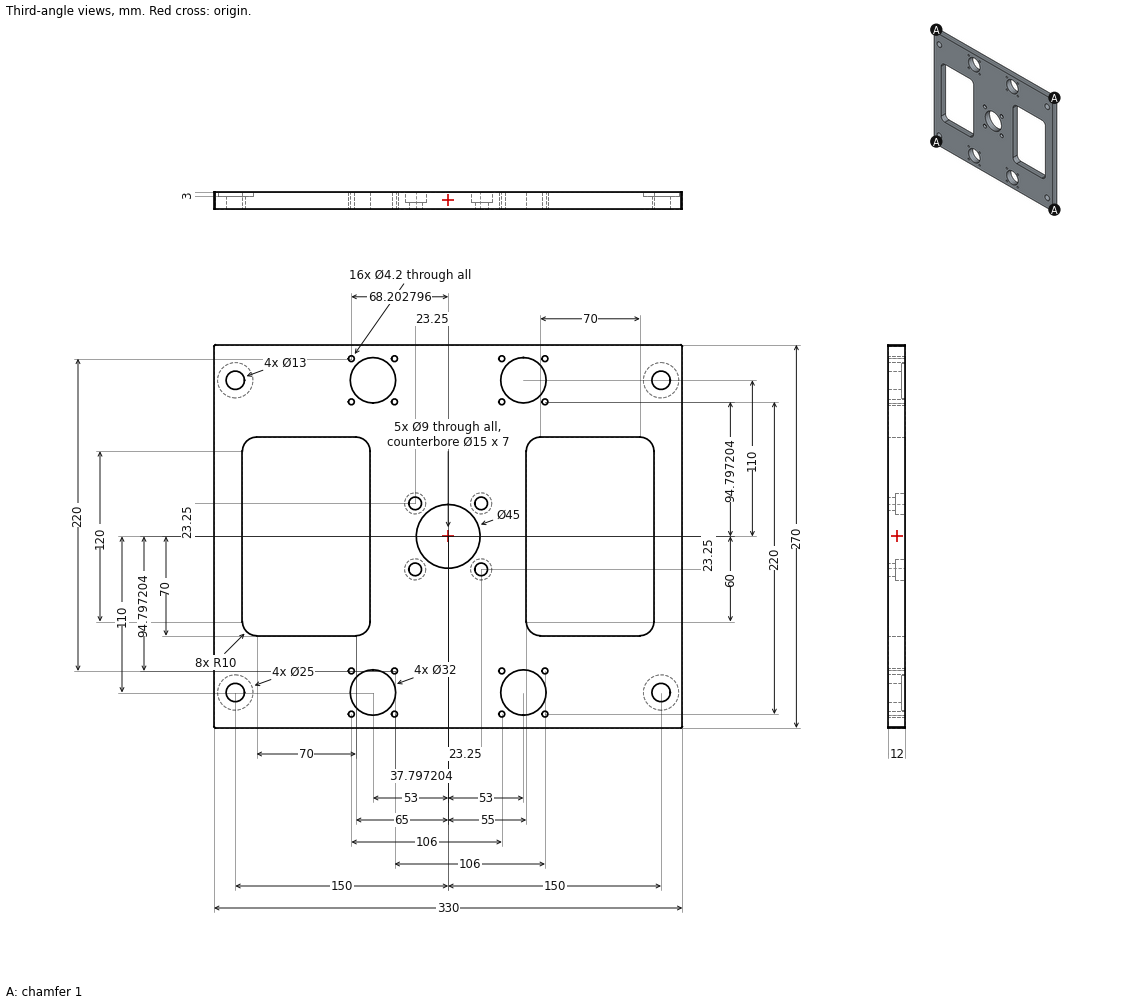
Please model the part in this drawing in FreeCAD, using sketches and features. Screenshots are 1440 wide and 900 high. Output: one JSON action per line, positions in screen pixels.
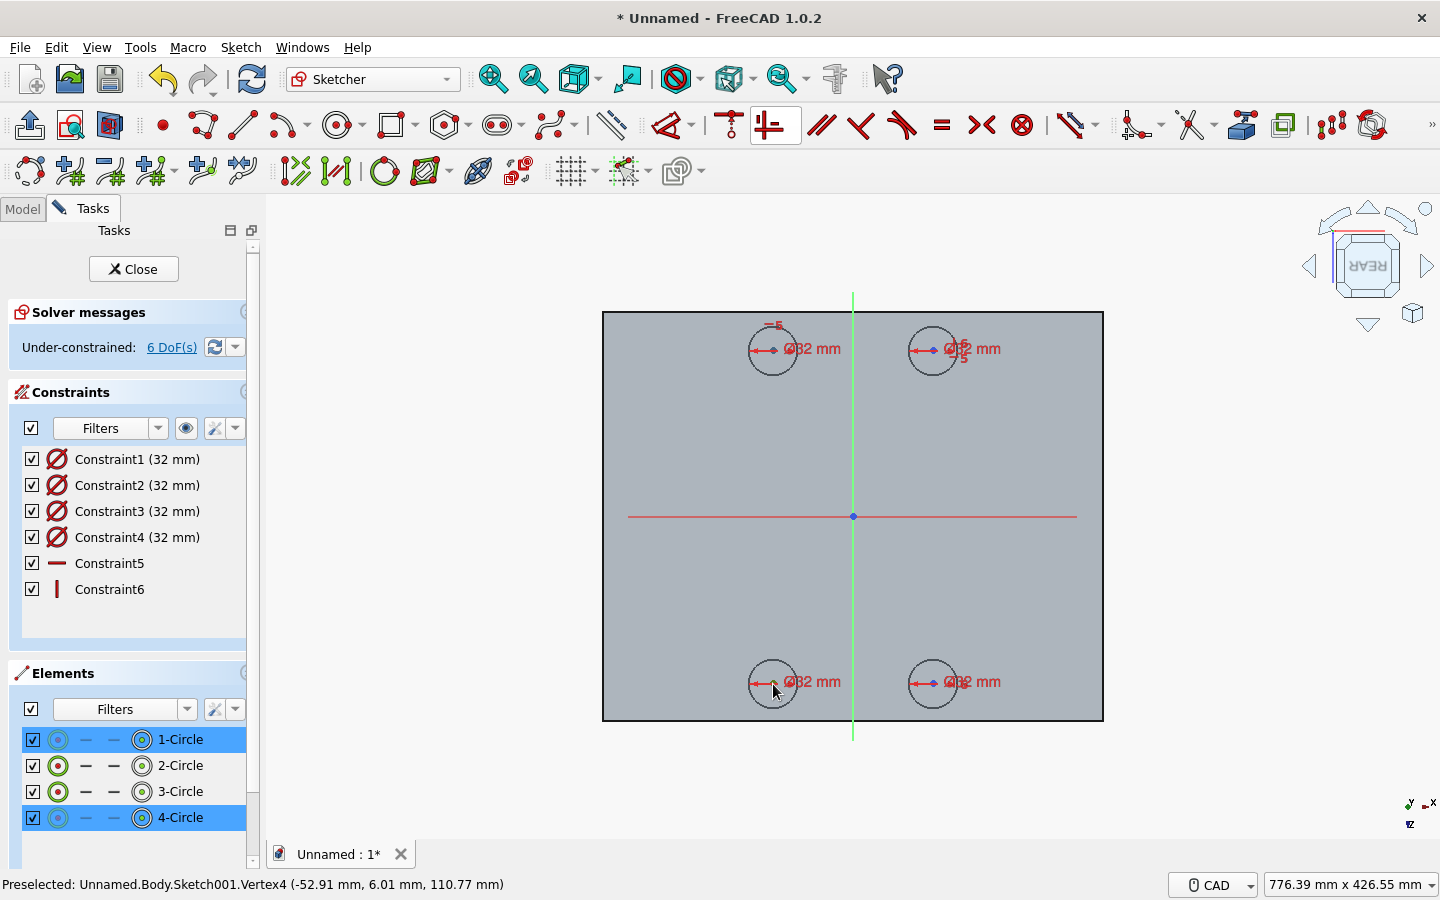
{"action": "left_click", "coordinate": [796, 126]}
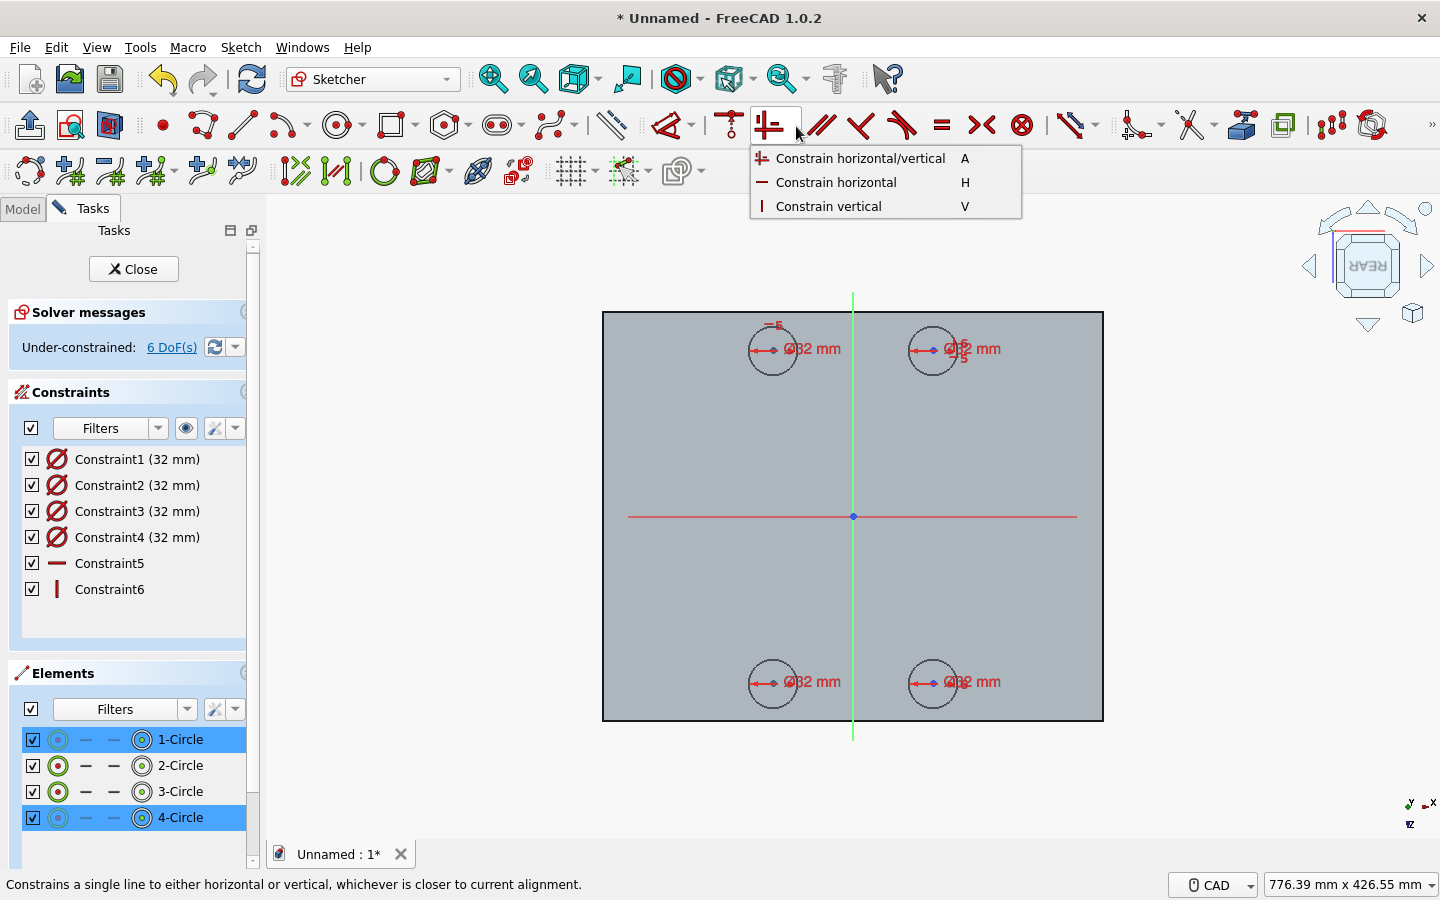
{"action": "left_click", "coordinate": [886, 206]}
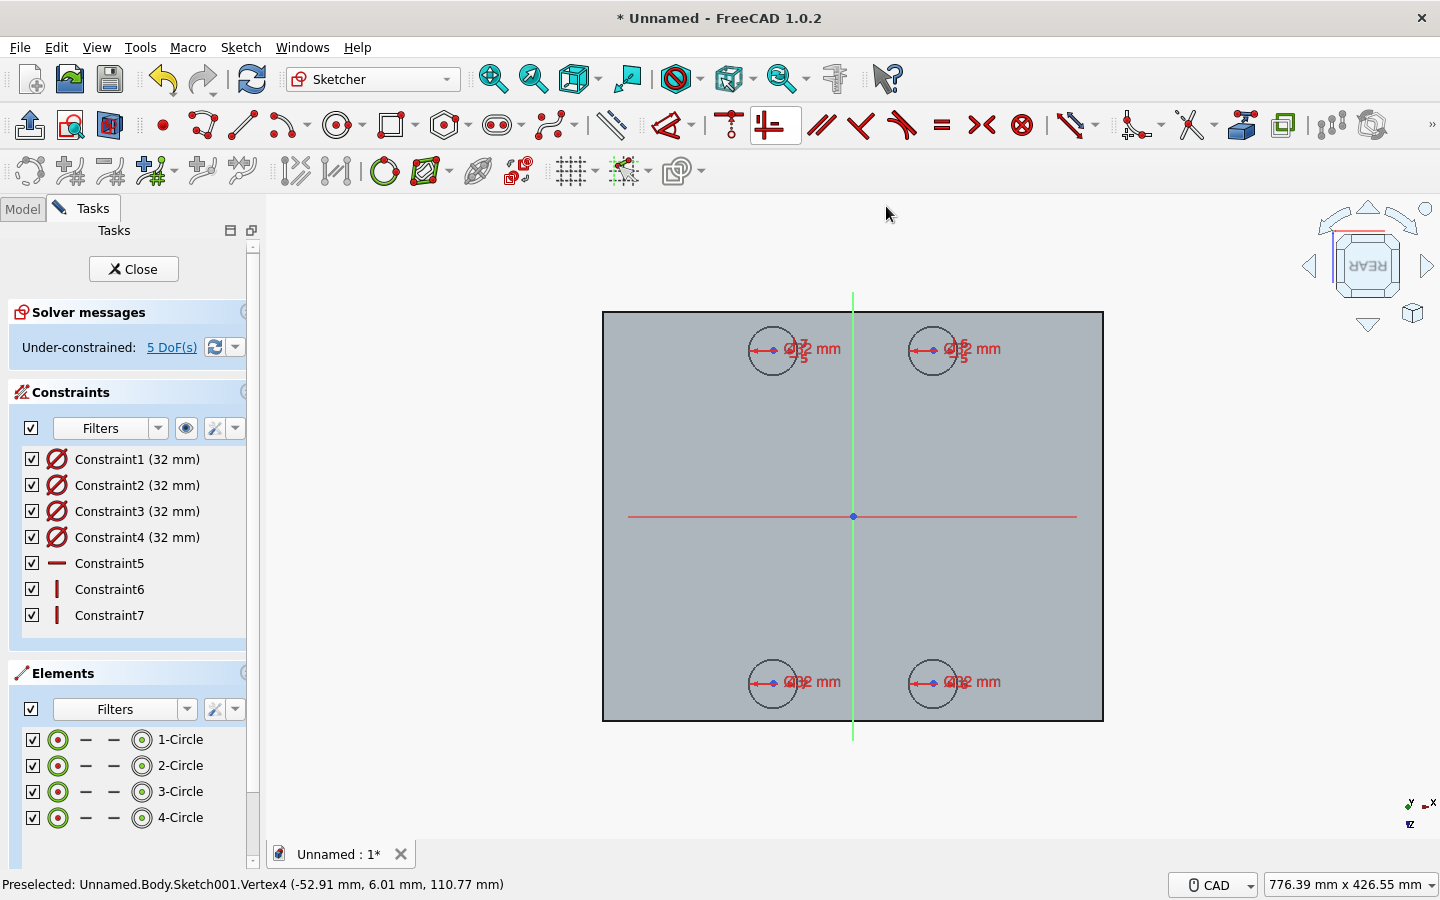
{"action": "left_click", "coordinate": [933, 684]}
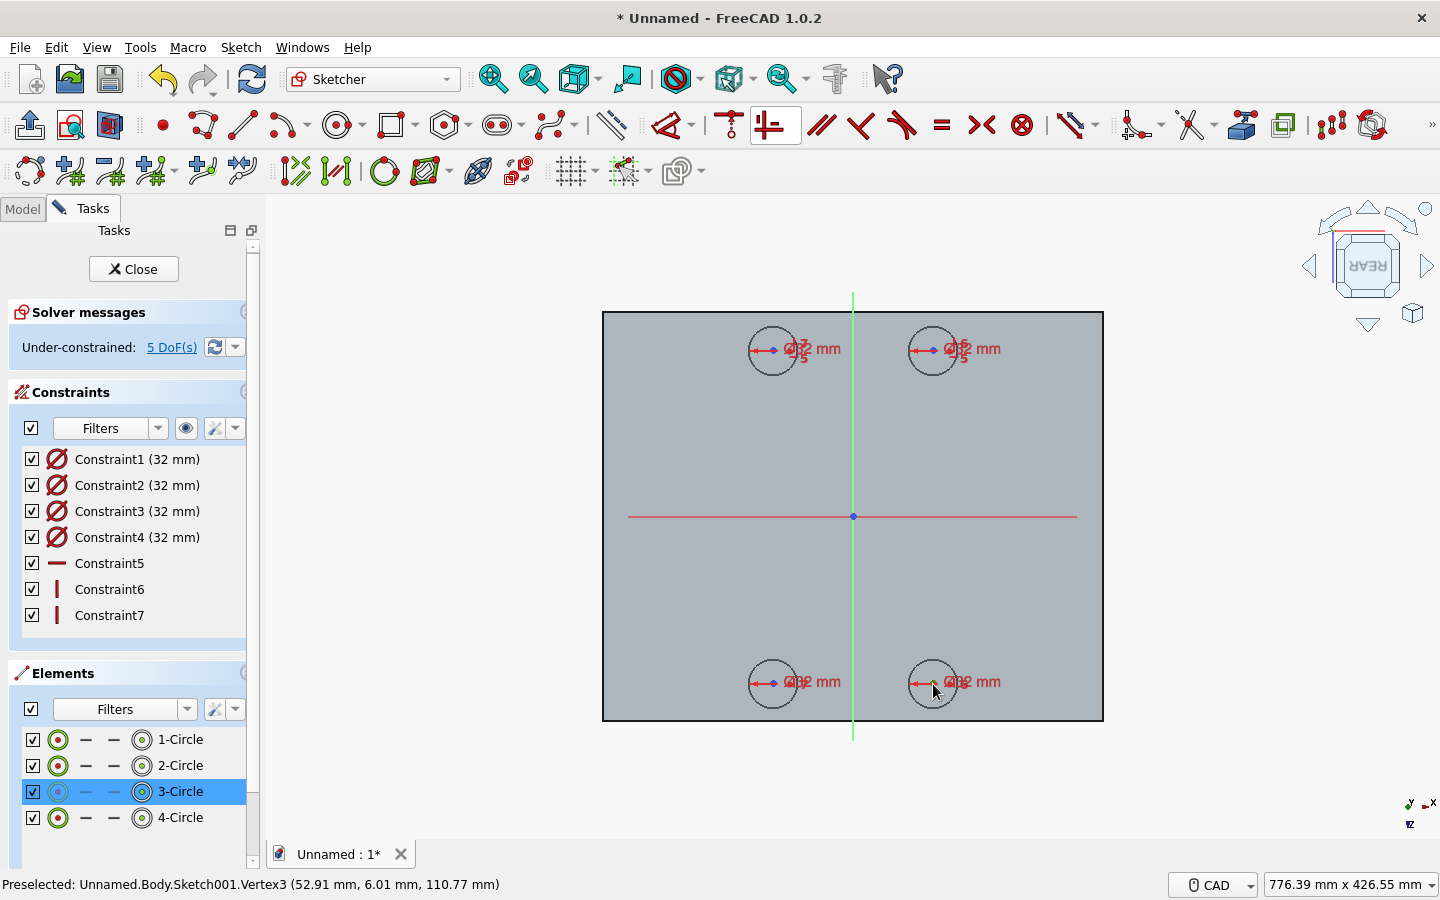
{"action": "left_click", "coordinate": [773, 684]}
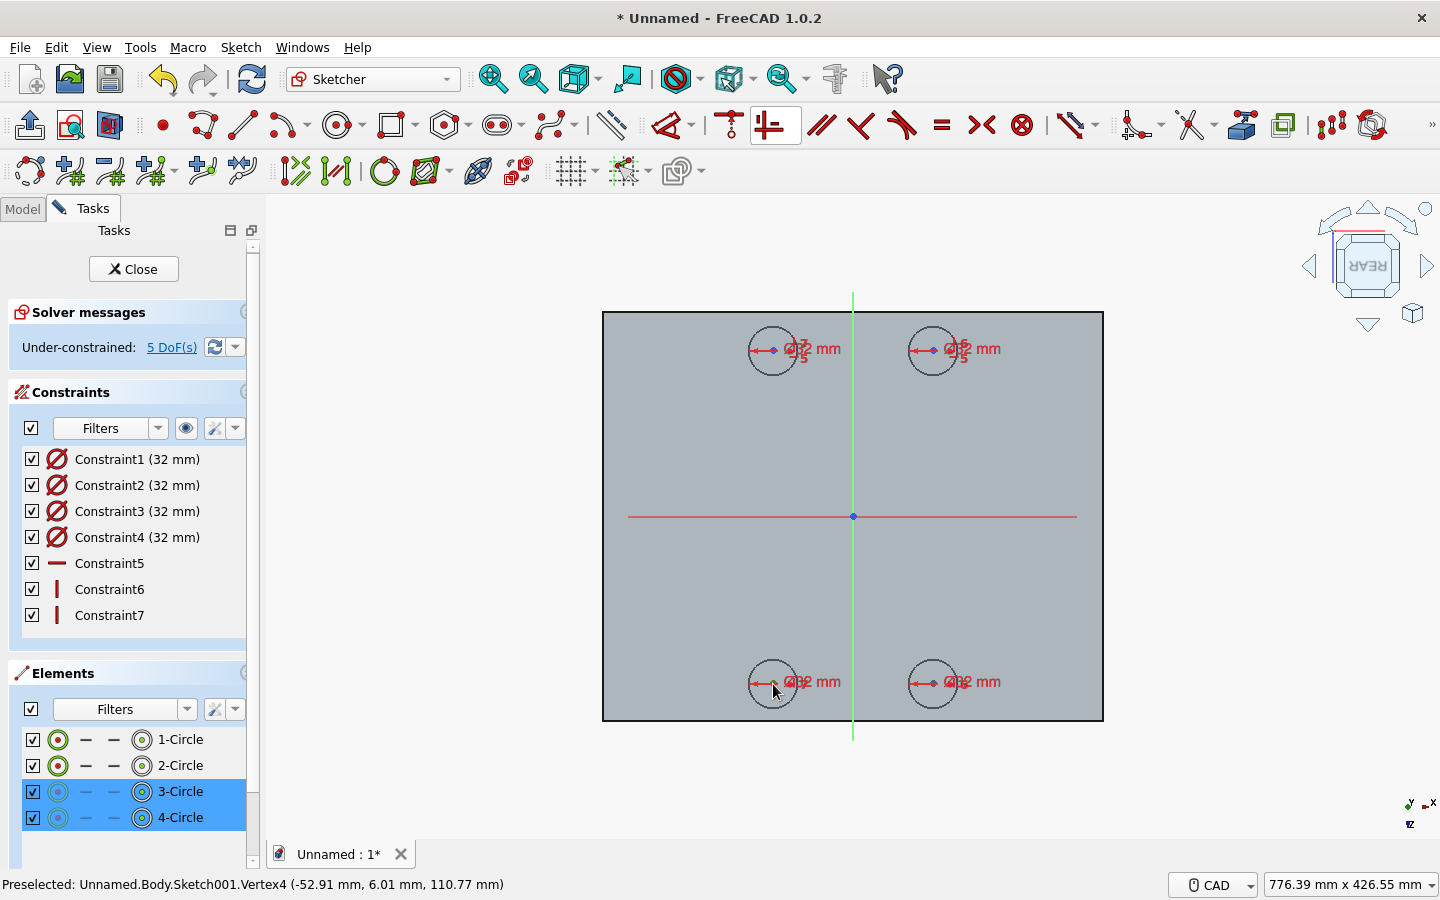
{"action": "left_click", "coordinate": [796, 126]}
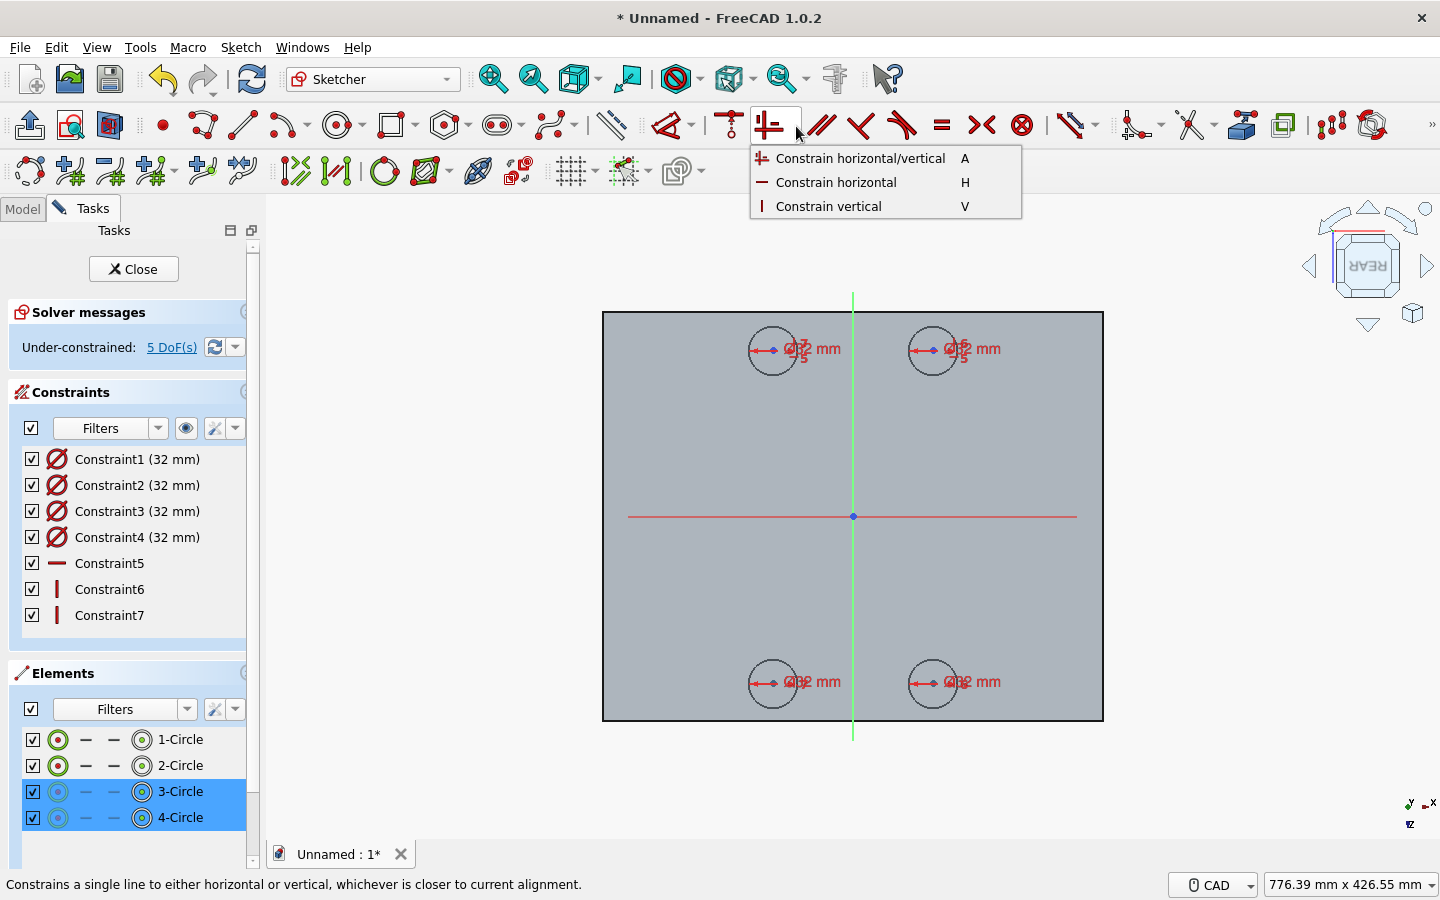
{"action": "left_click", "coordinate": [886, 182]}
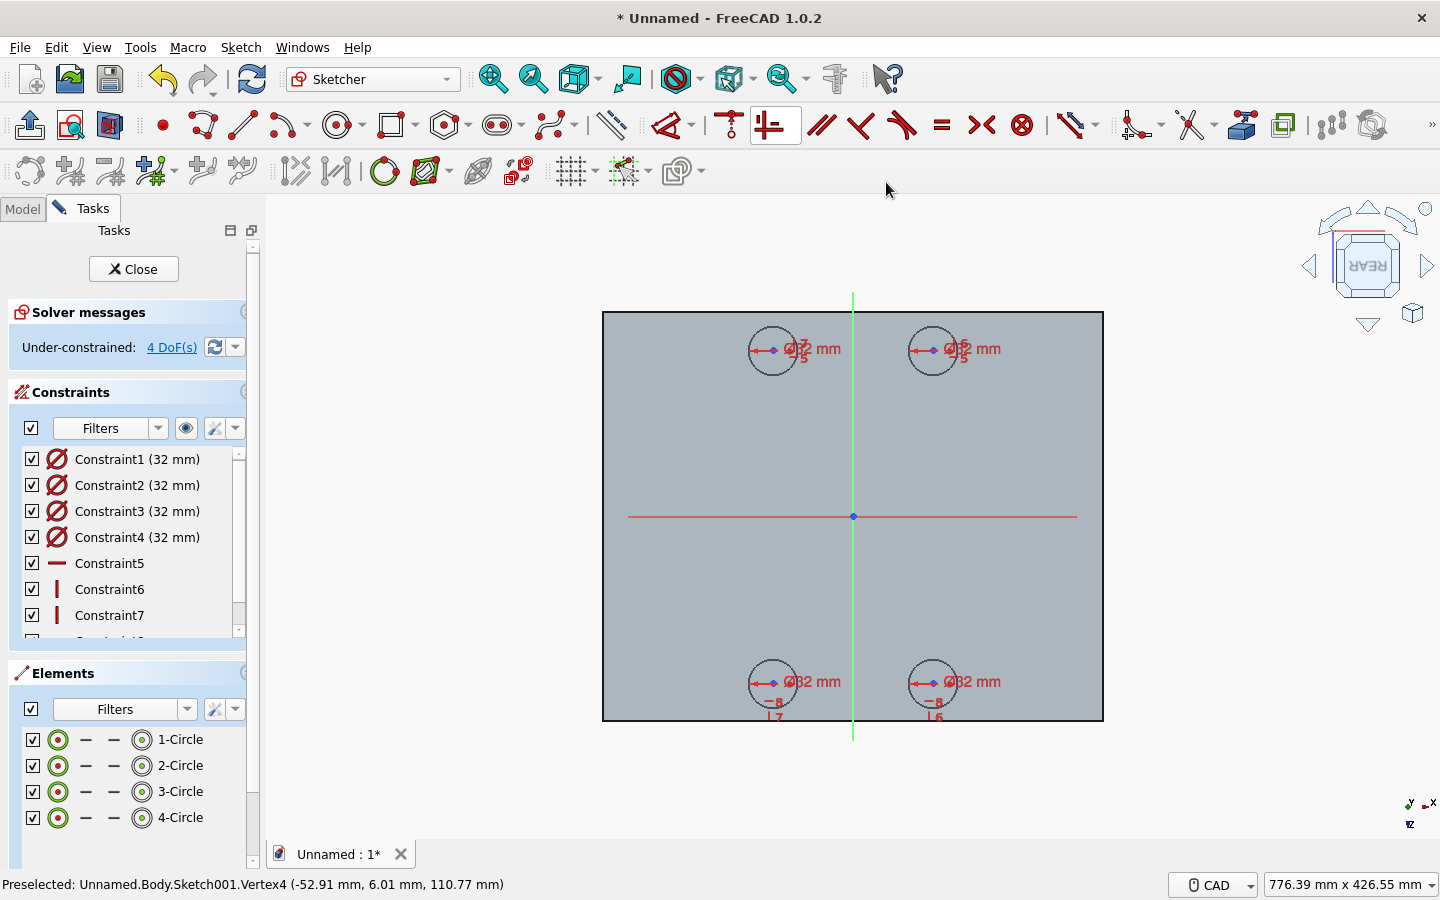
{"action": "key", "text": "d"}